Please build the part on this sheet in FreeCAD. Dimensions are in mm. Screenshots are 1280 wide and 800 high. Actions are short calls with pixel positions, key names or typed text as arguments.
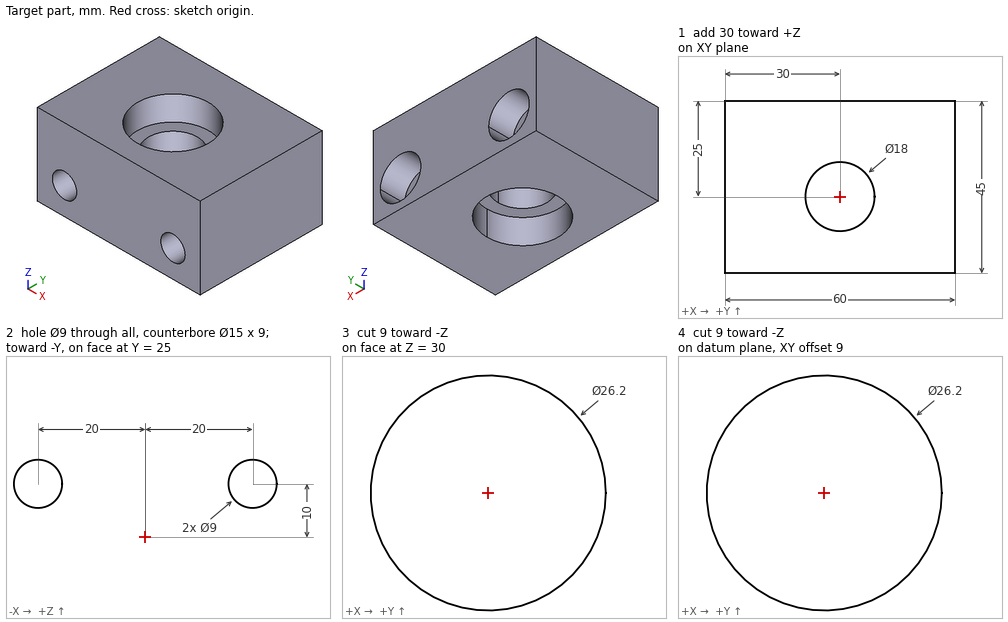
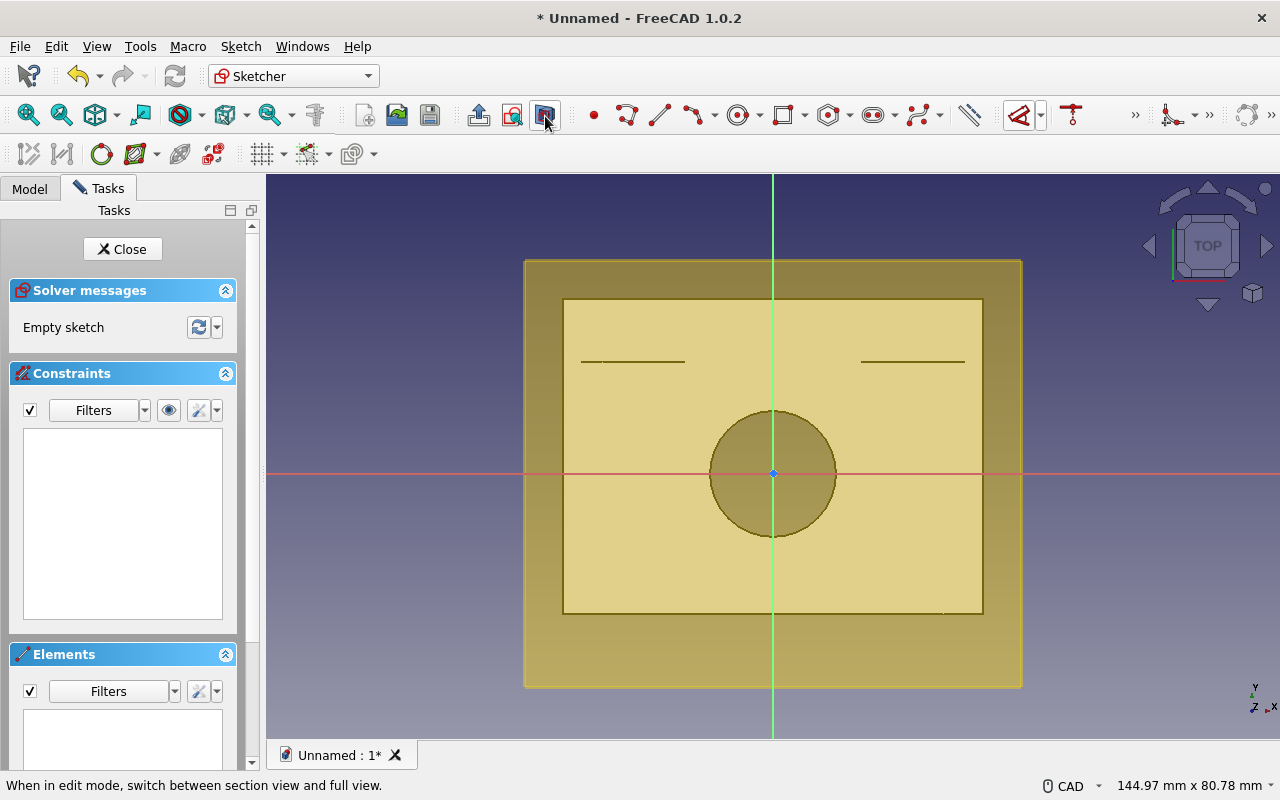
scroll(856, 495, up, 3)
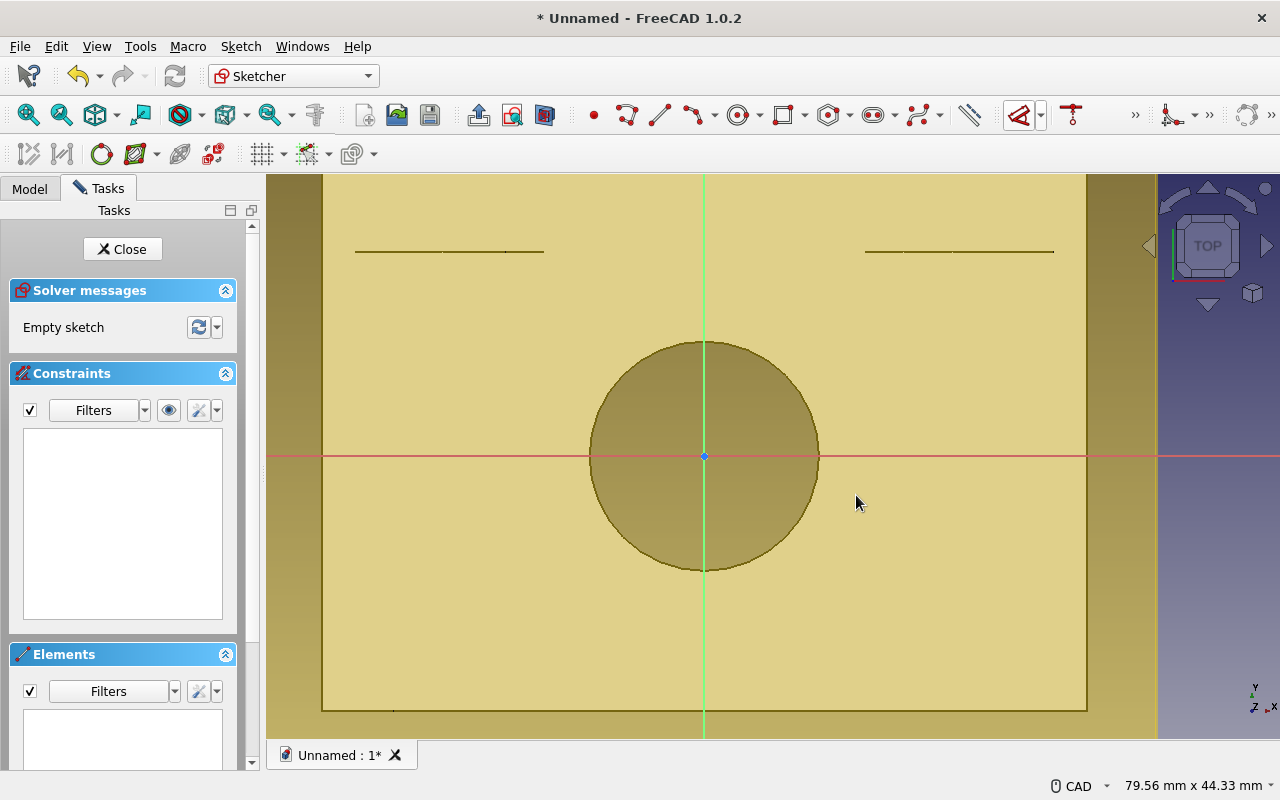
click(738, 116)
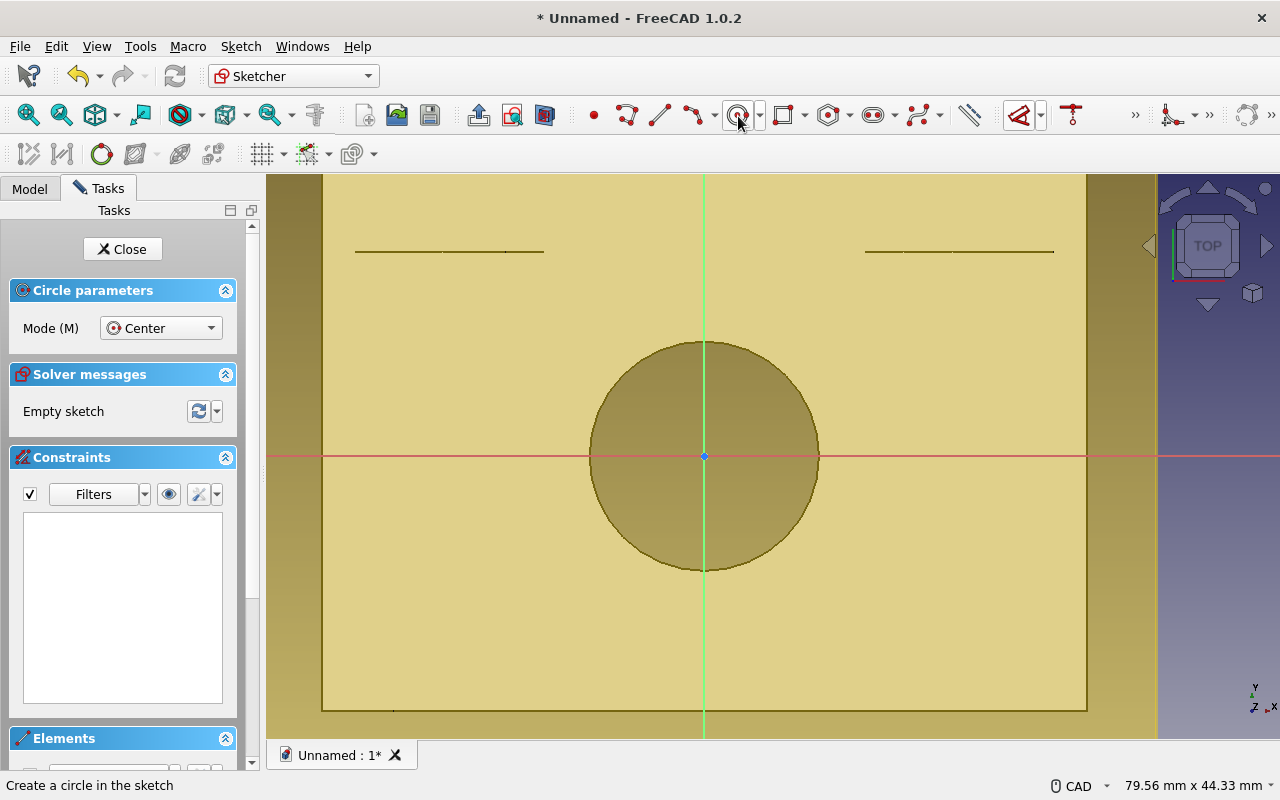
click(704, 456)
move(822, 338)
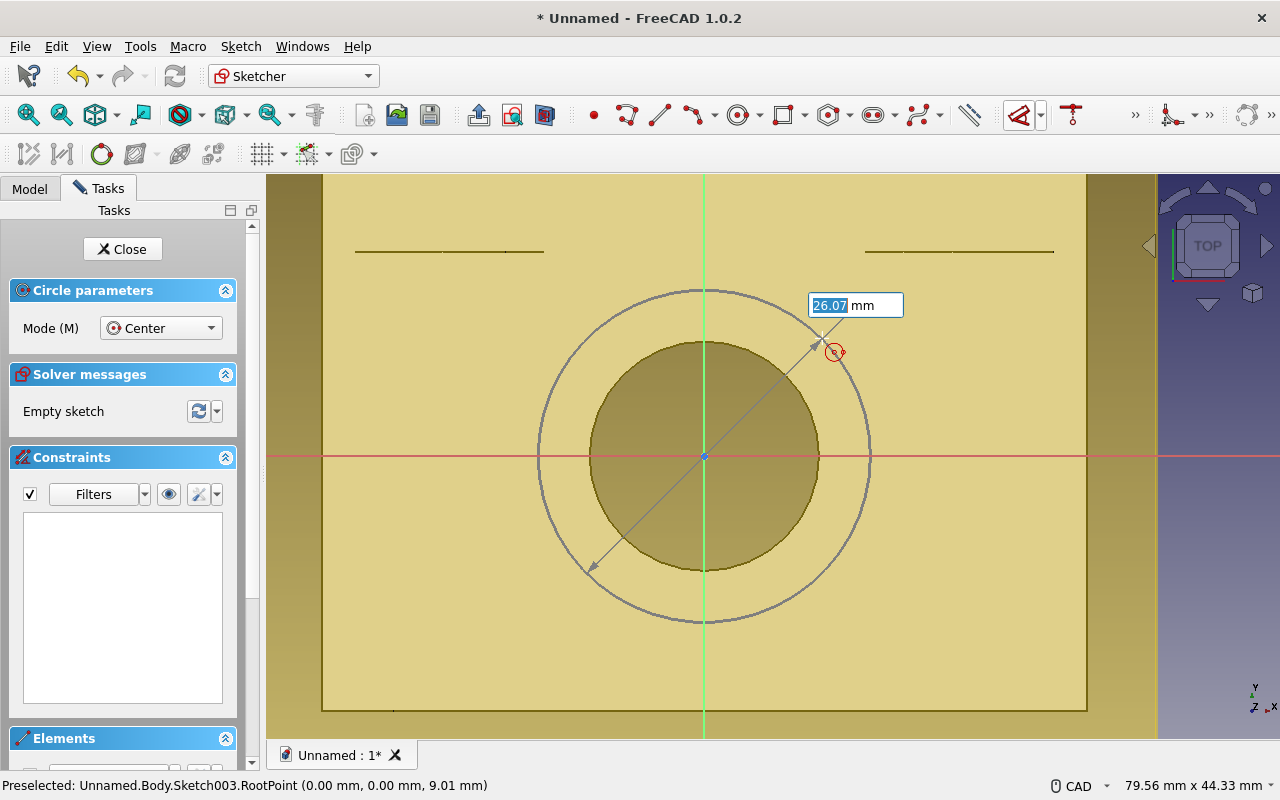
text(26.2)
key(Return)
key(Escape)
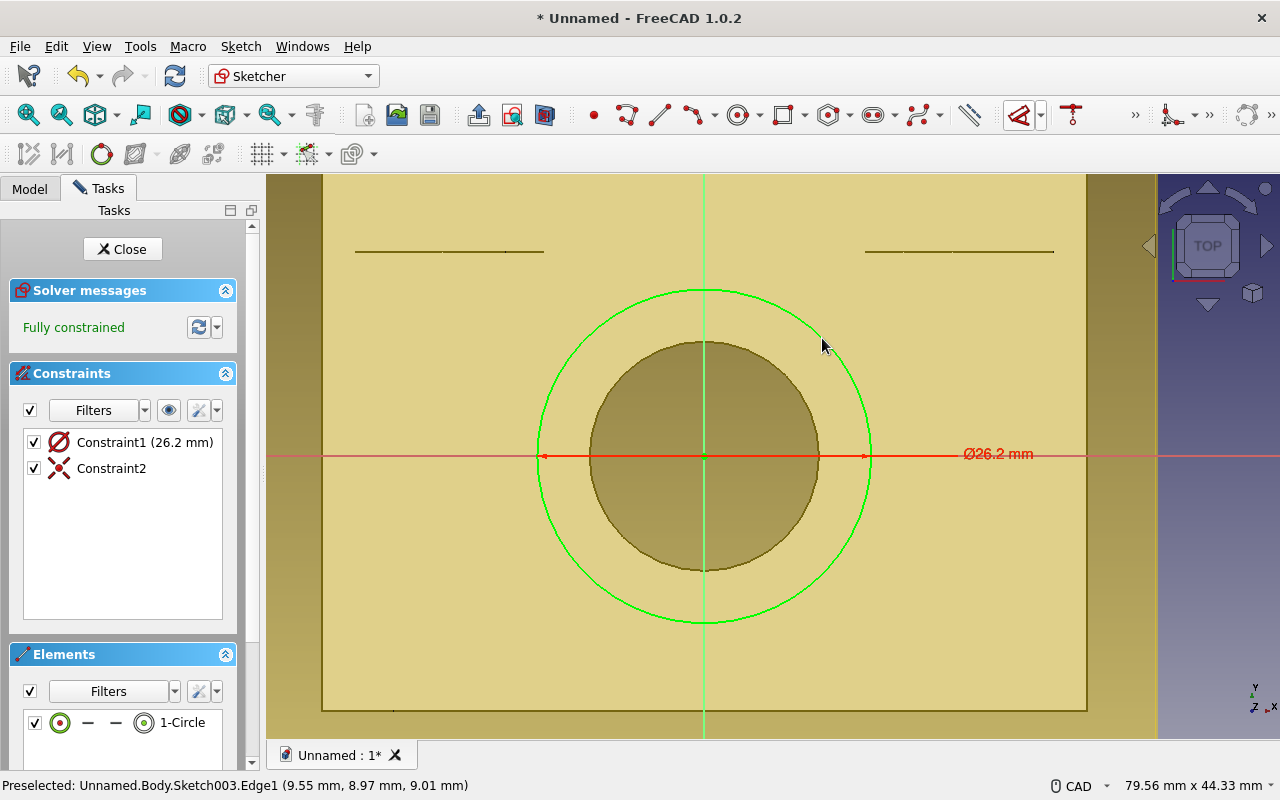
click(123, 249)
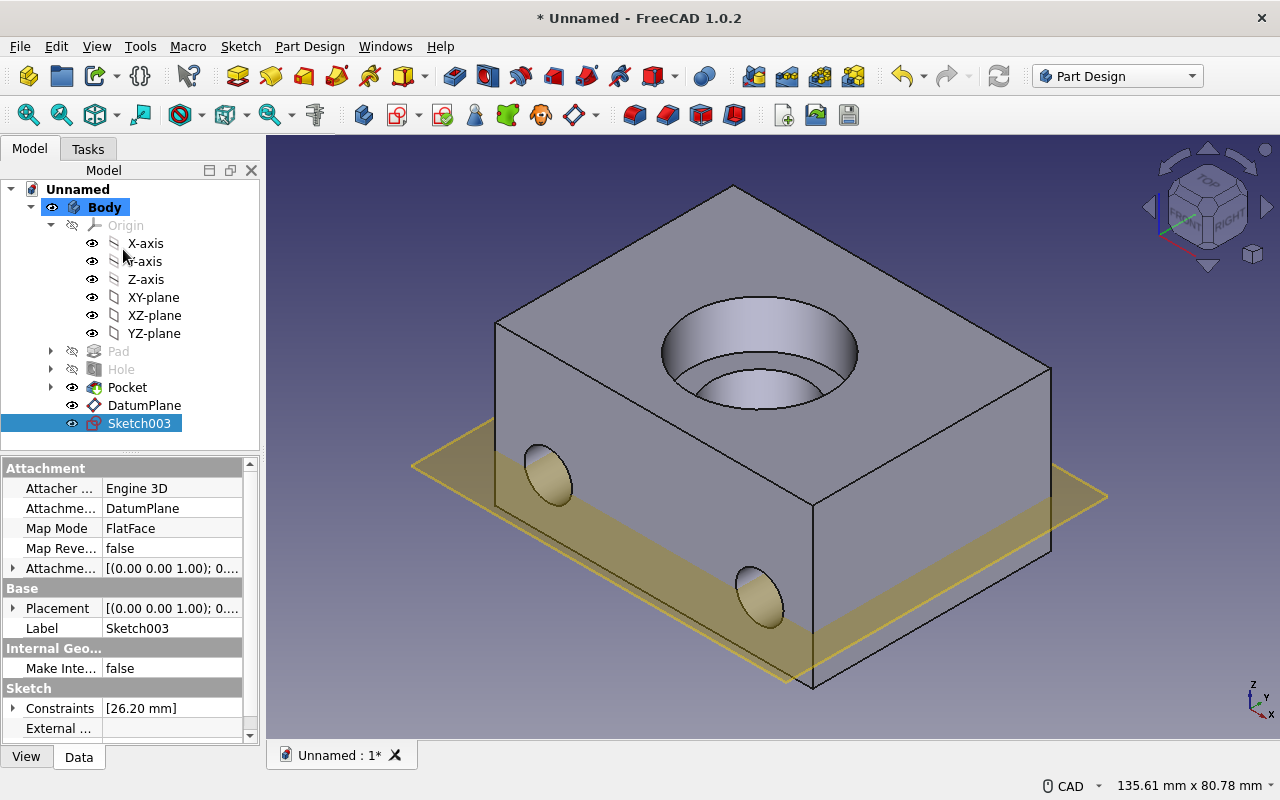
click(455, 76)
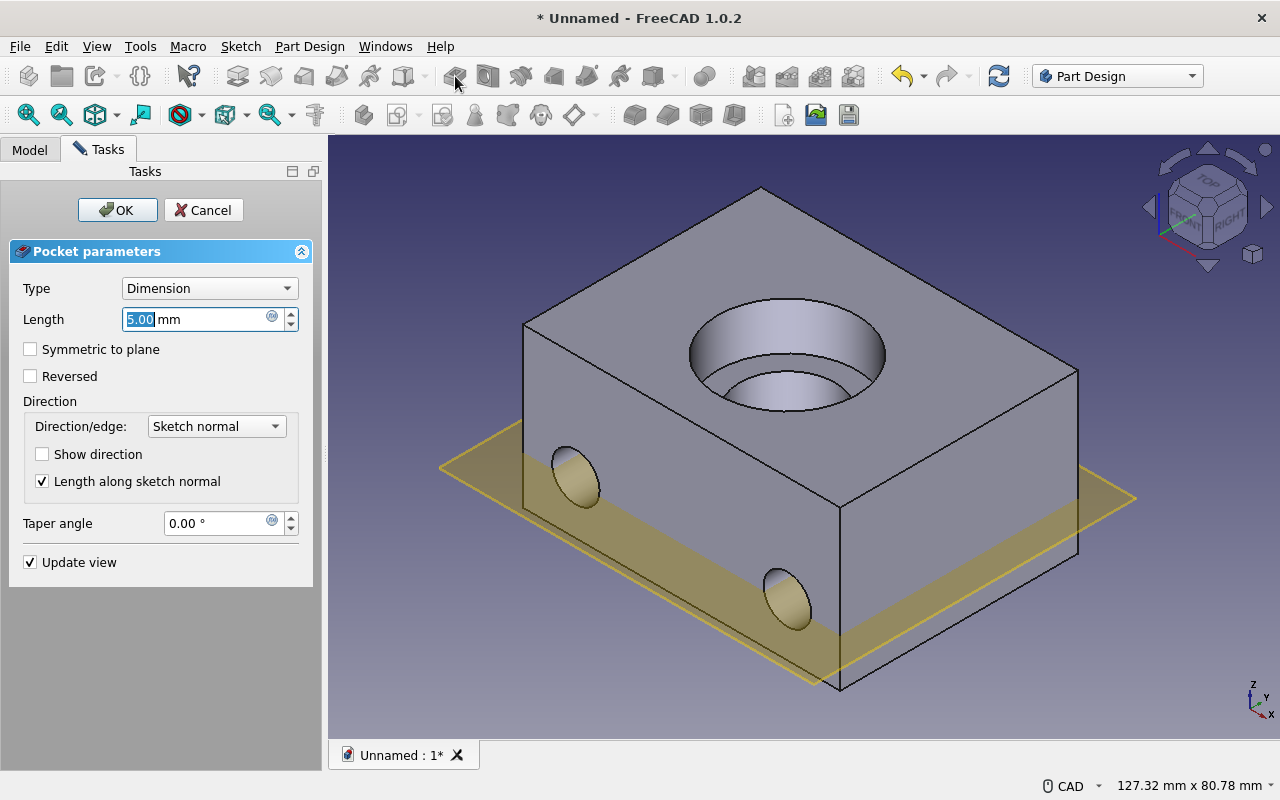
text(9)
key(Tab)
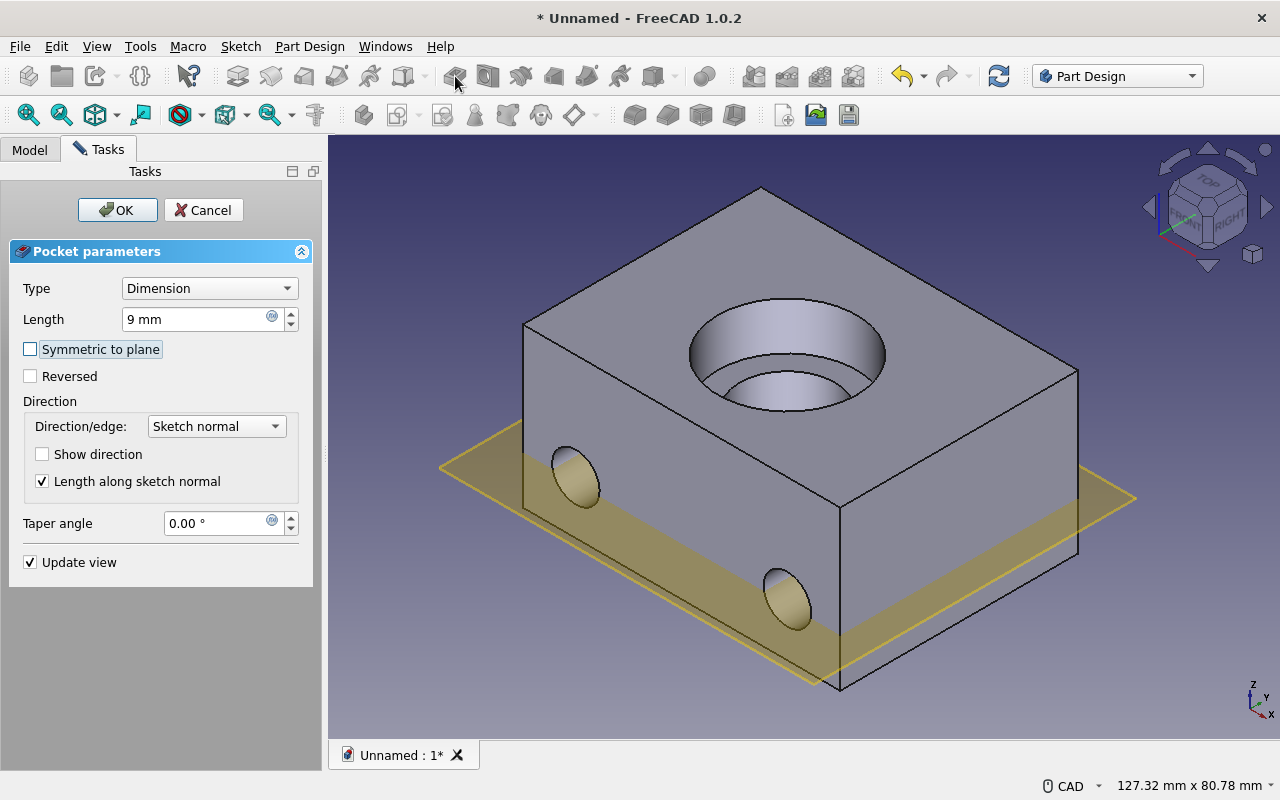
click(118, 210)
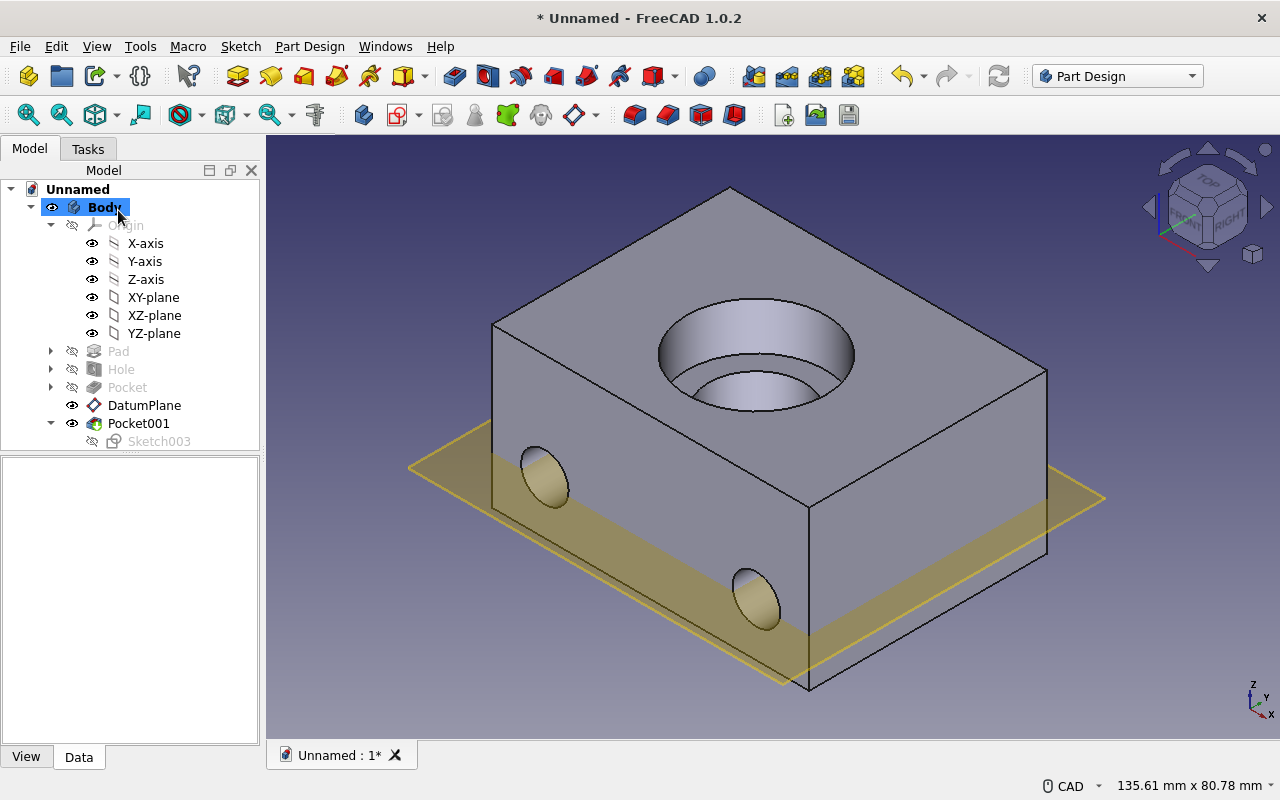
click(117, 405)
key(space)